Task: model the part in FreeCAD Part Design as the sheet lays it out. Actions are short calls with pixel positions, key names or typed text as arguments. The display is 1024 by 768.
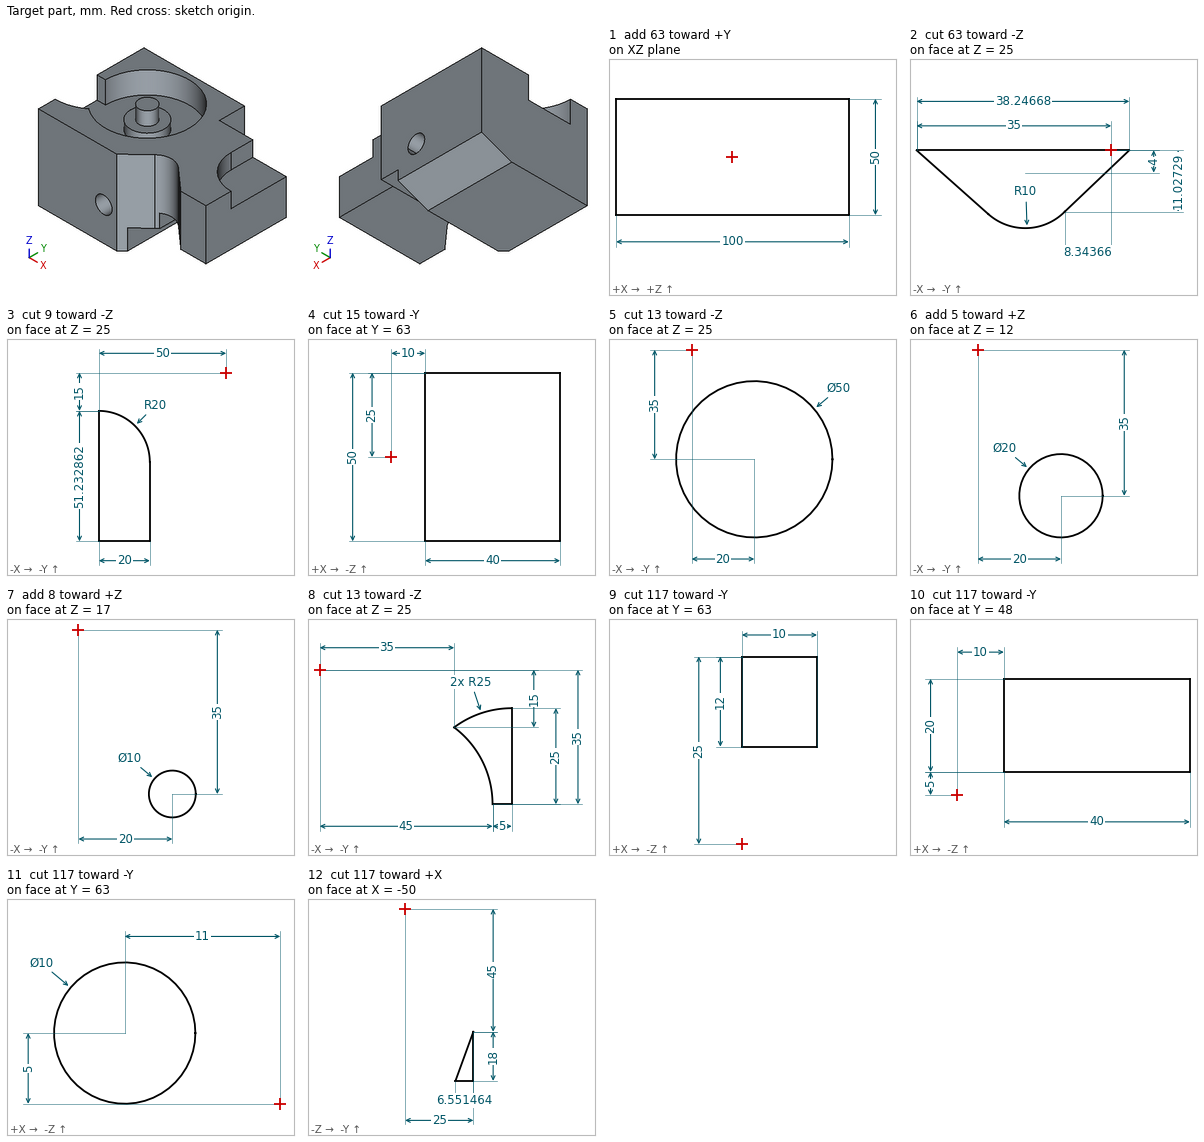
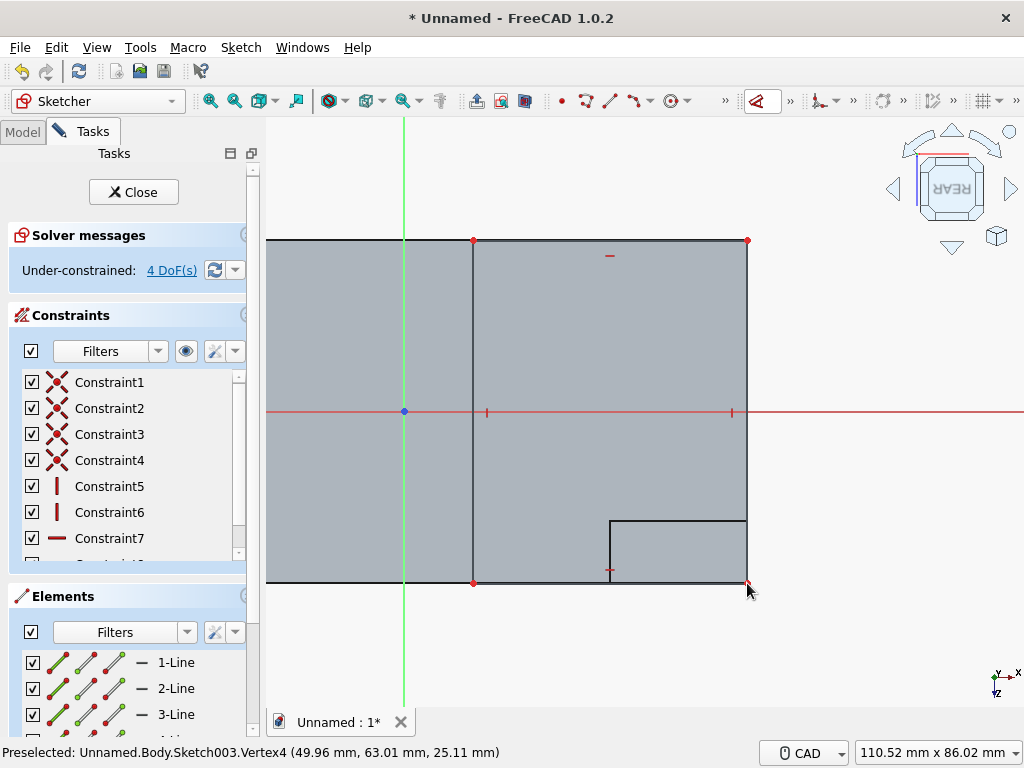
click(473, 344)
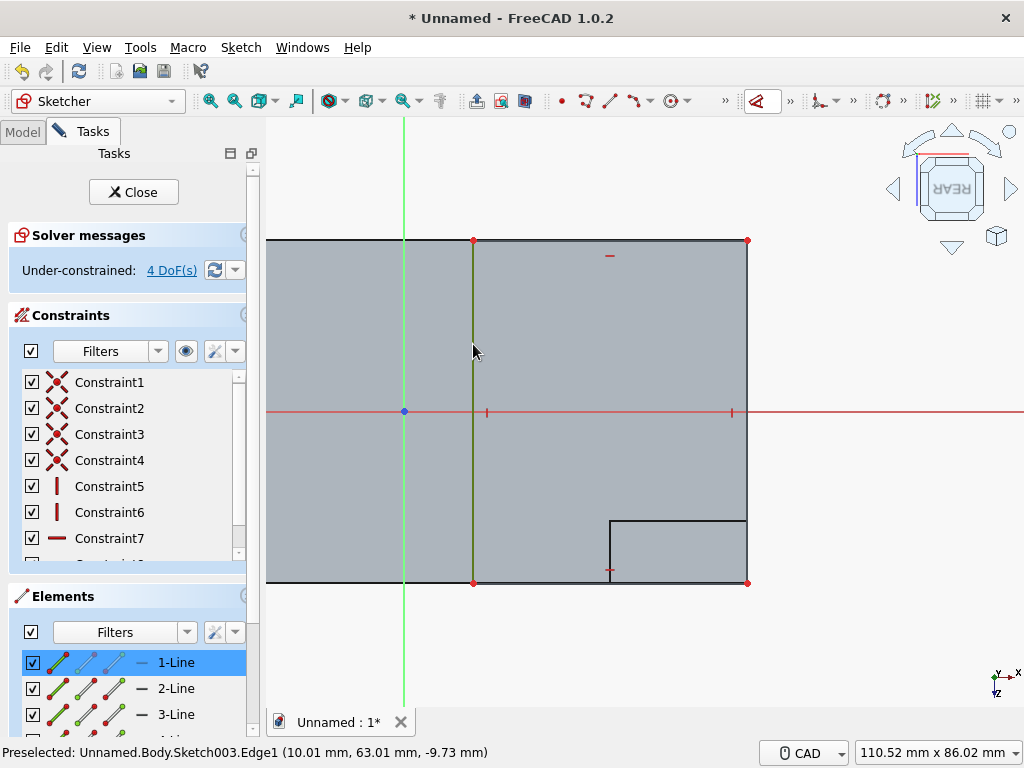
key(i)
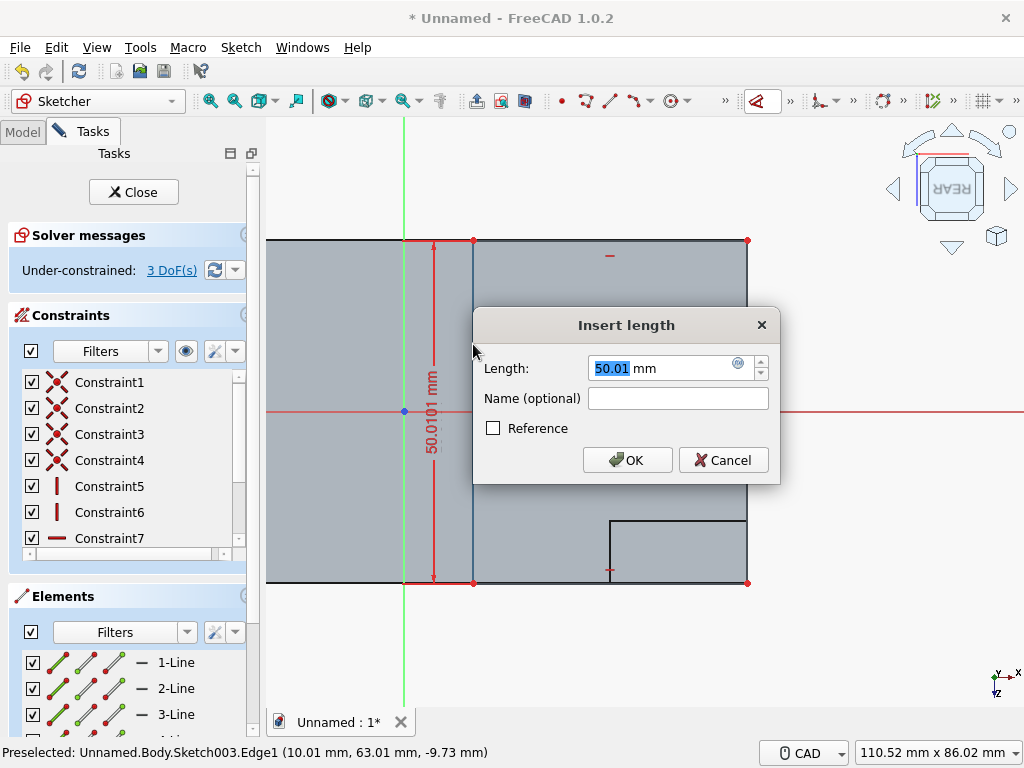
text(50)
key(Return)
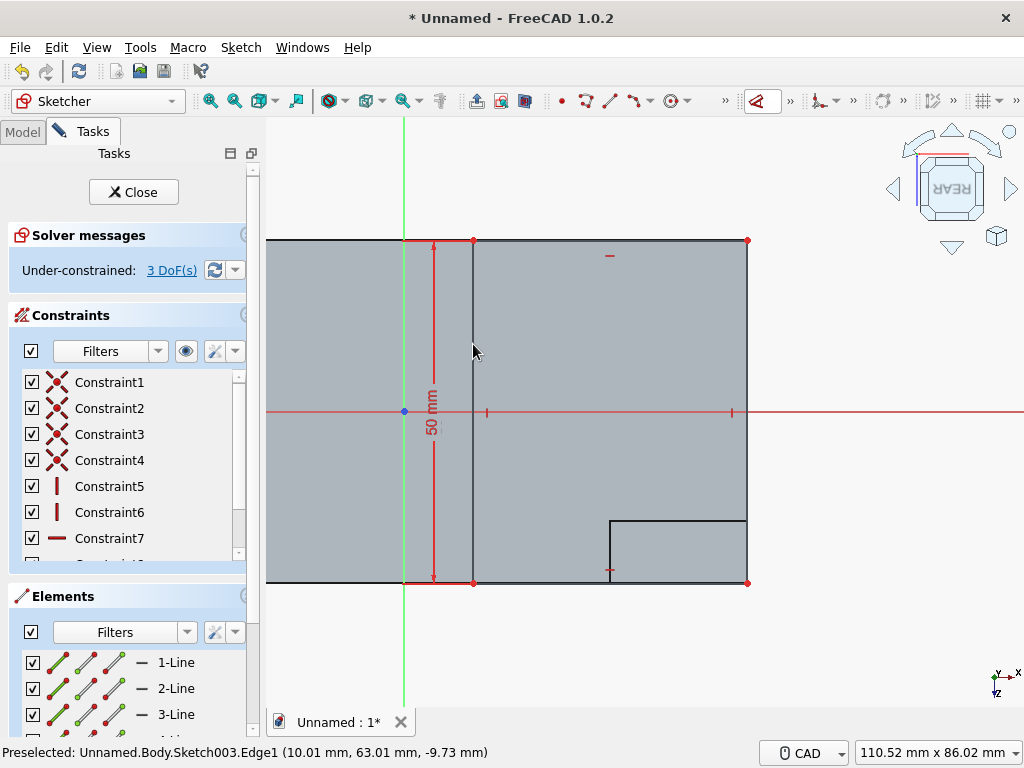
click(555, 584)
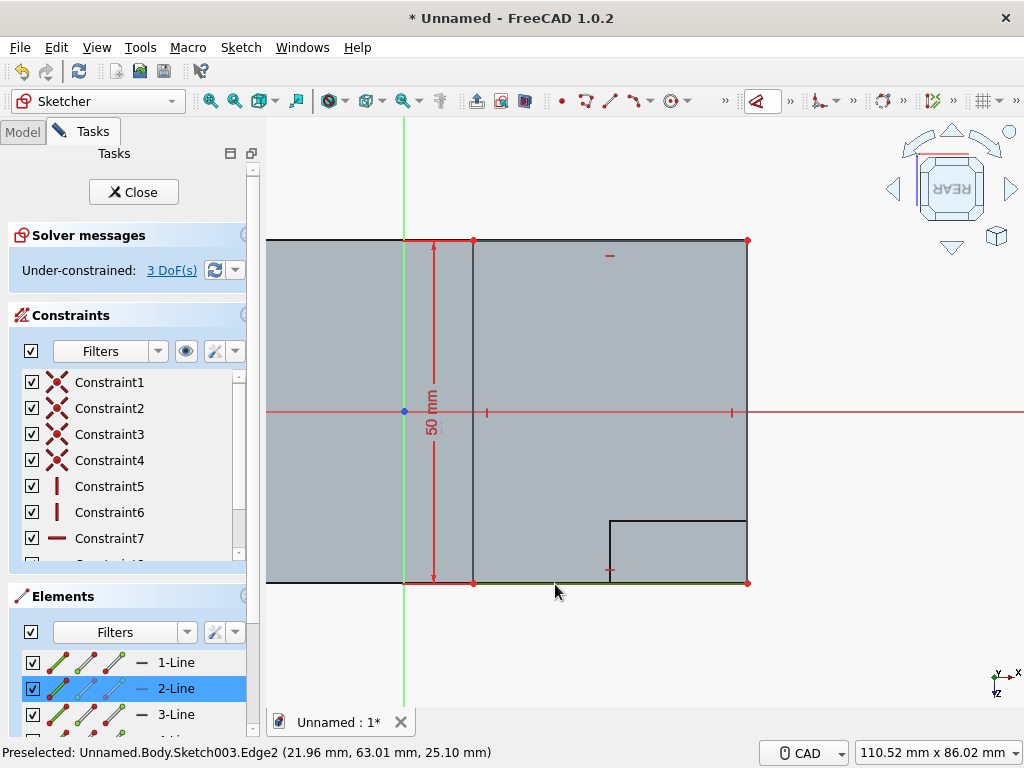
key(l)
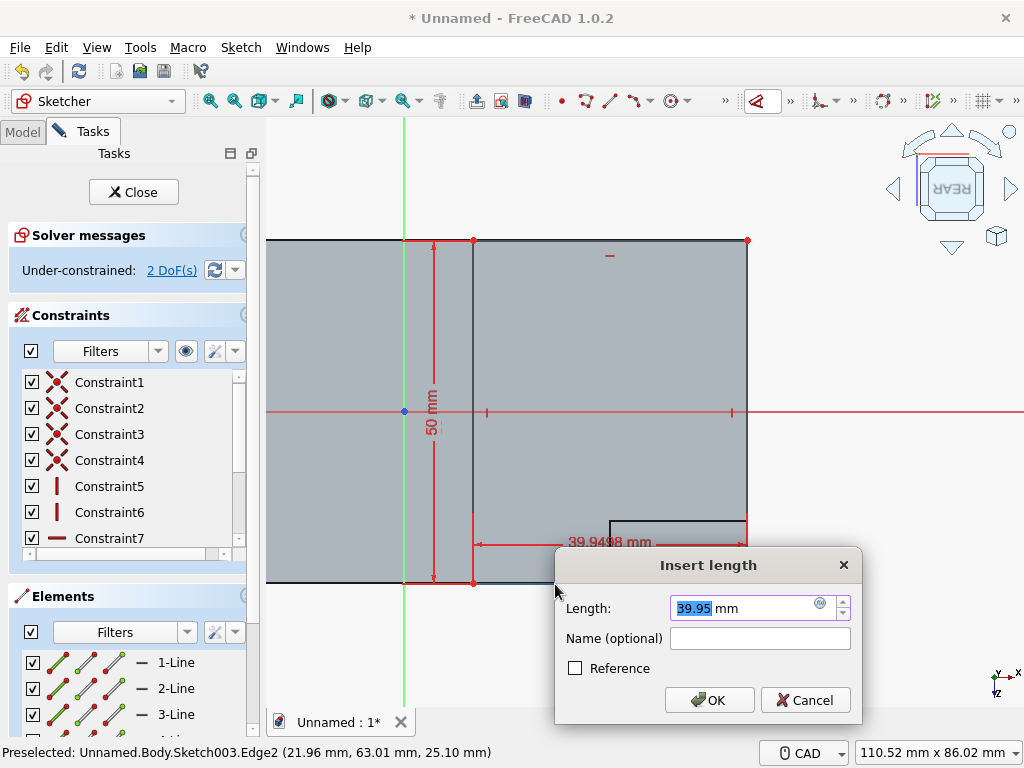
text(40)
key(Return)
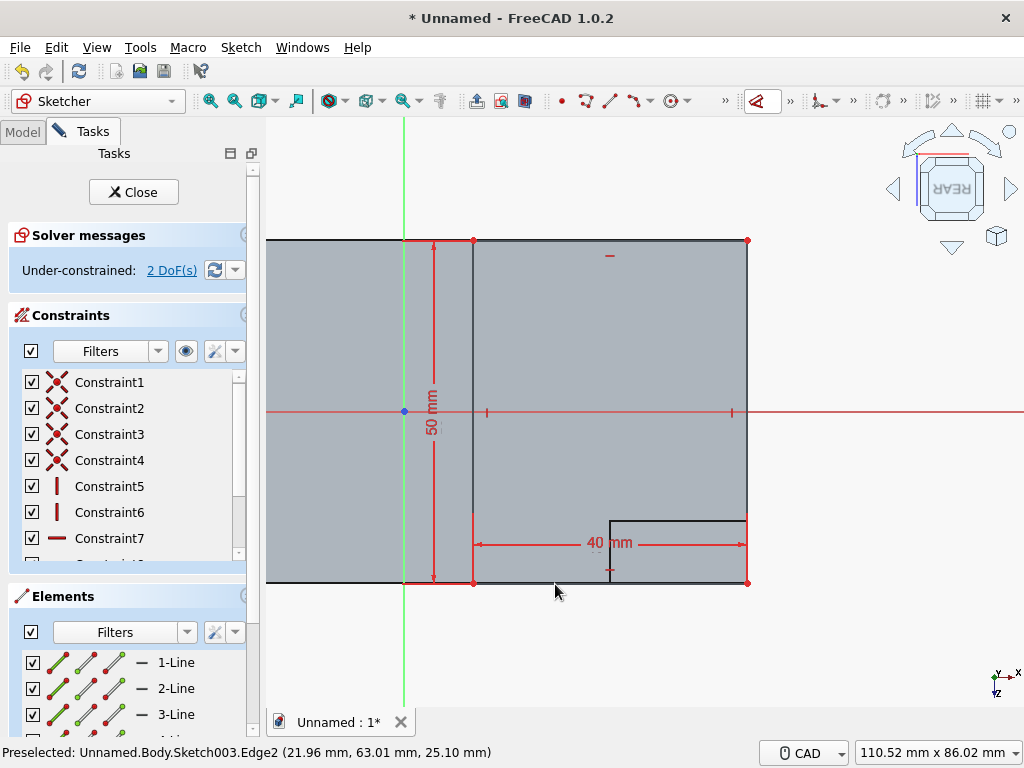
click(473, 241)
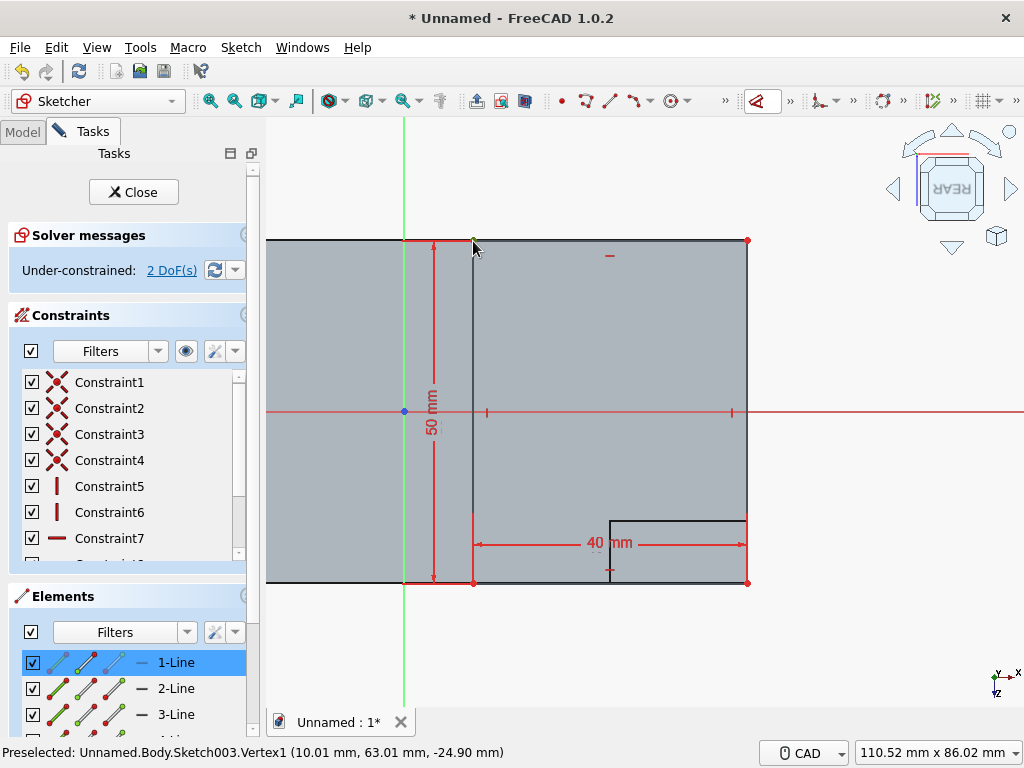
key(l)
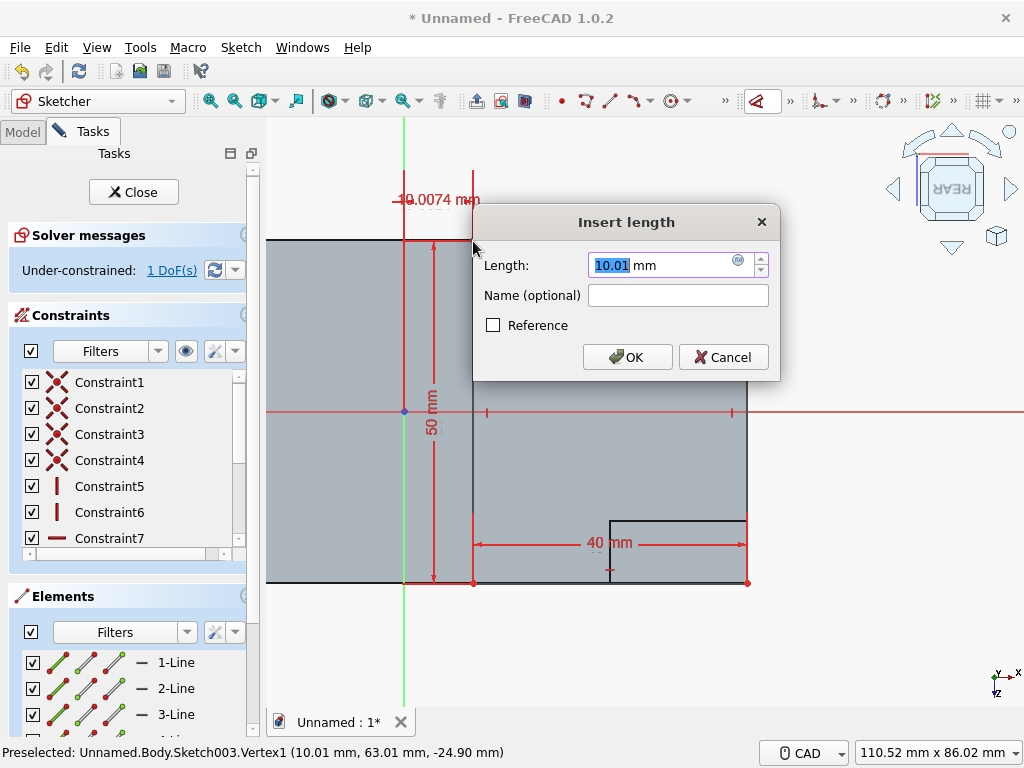
text(10)
key(Return)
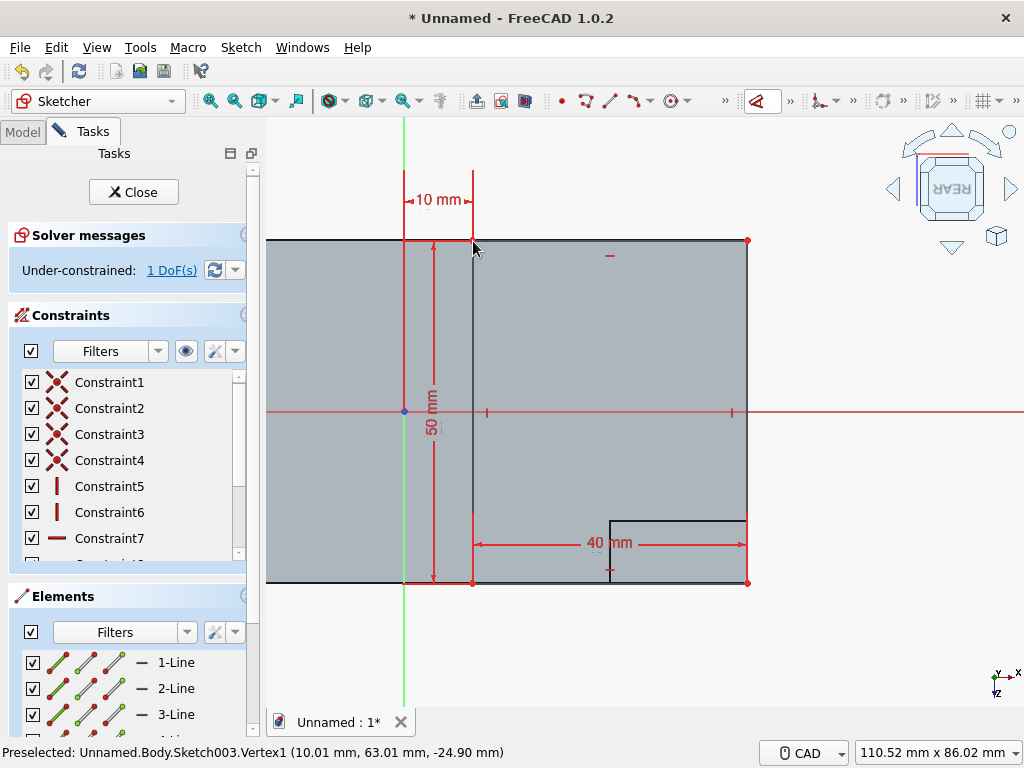
click(473, 241)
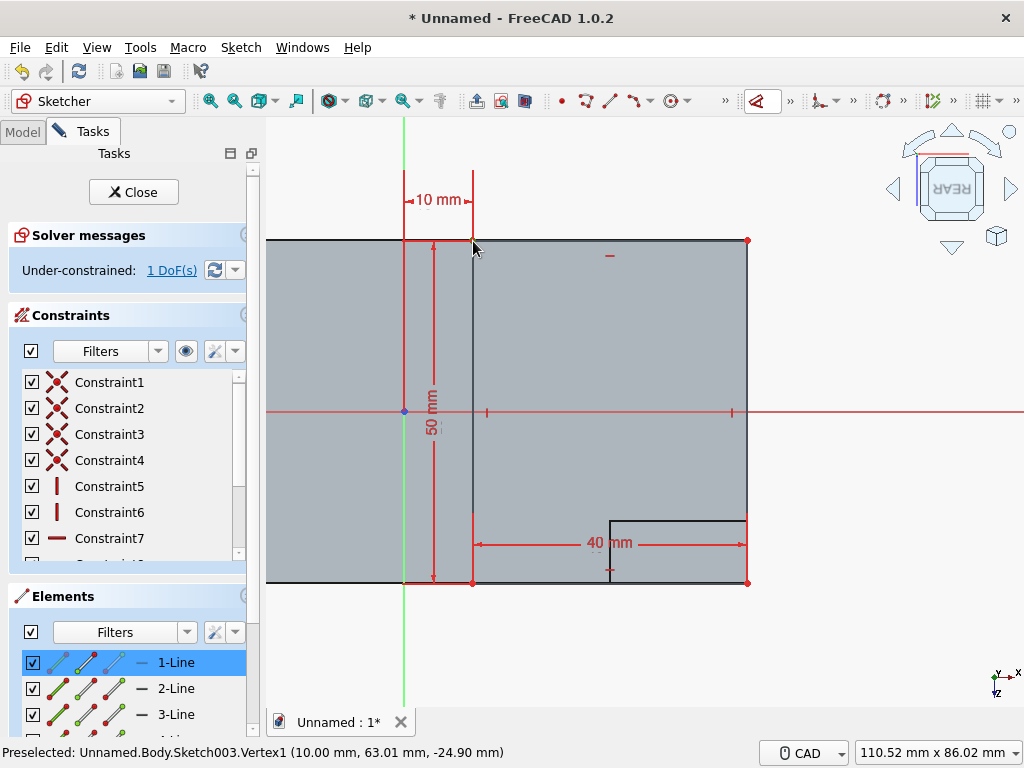
click(776, 102)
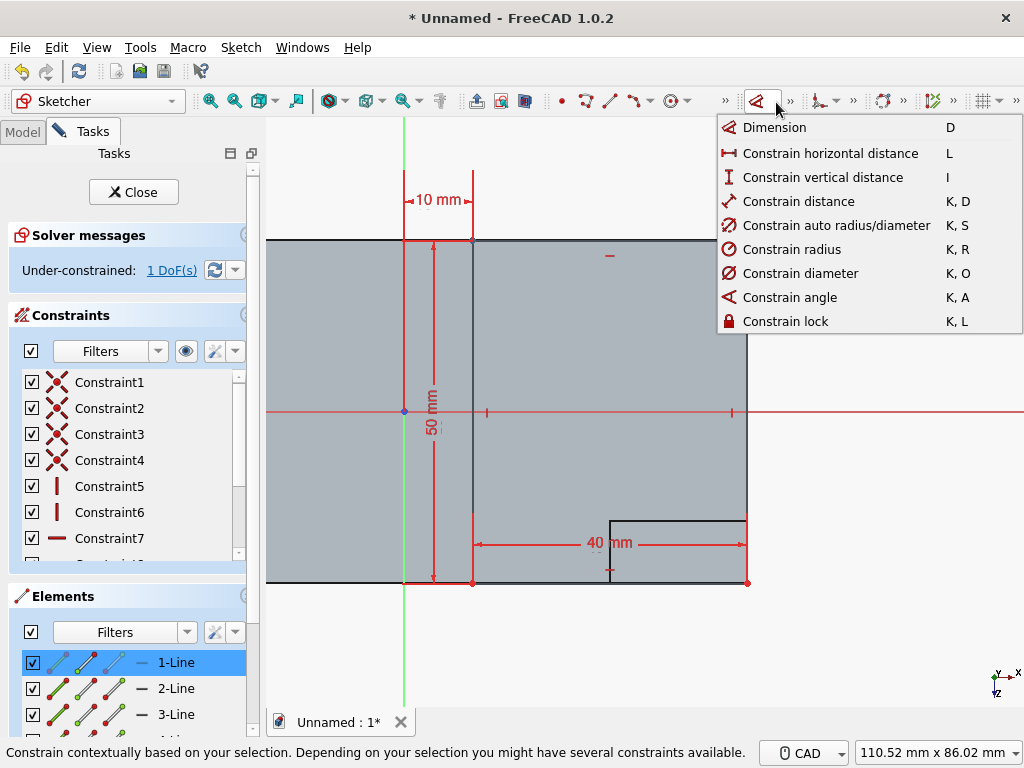
click(870, 177)